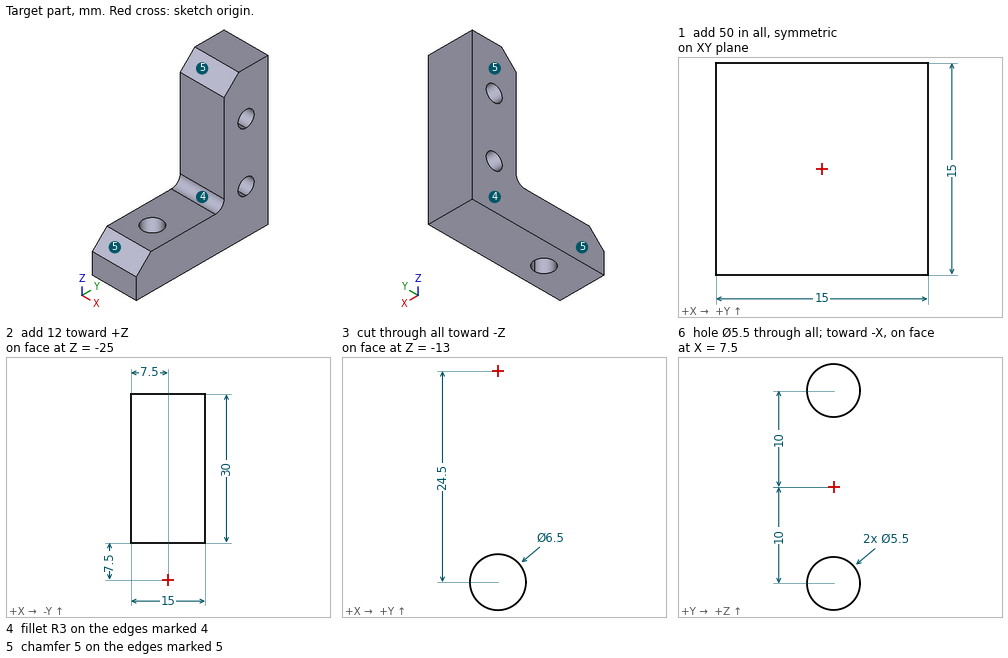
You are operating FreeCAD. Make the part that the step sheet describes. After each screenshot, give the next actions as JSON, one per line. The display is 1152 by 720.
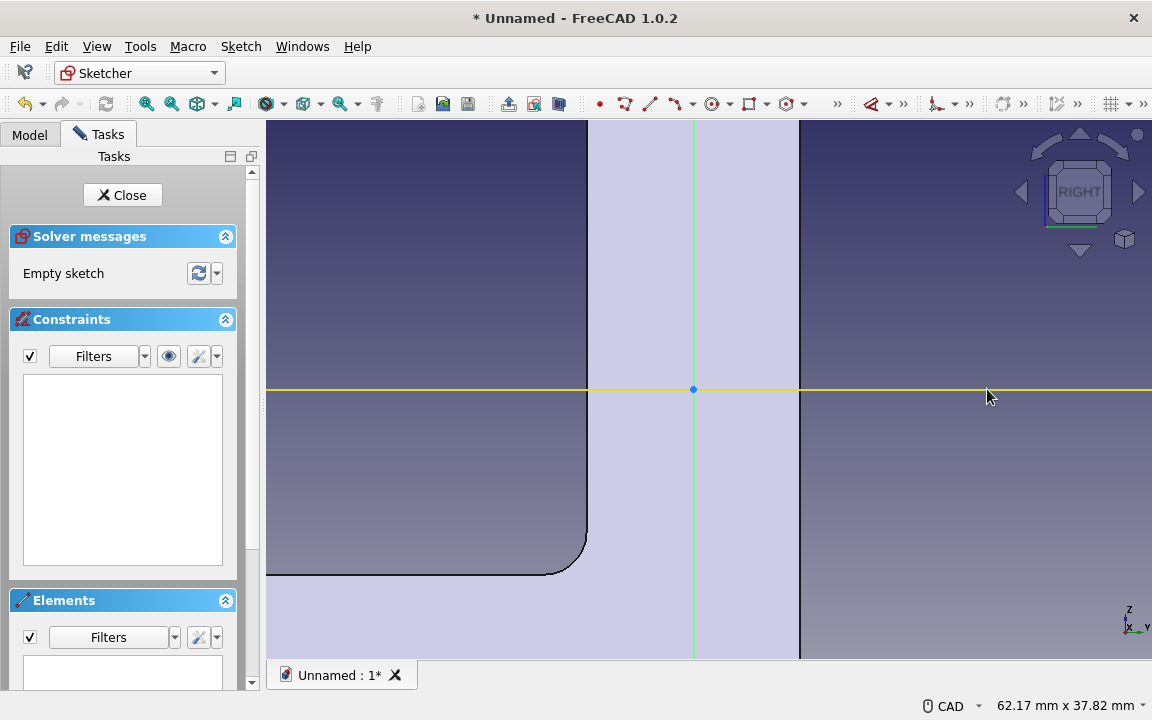
{"action": "key", "text": "g c"}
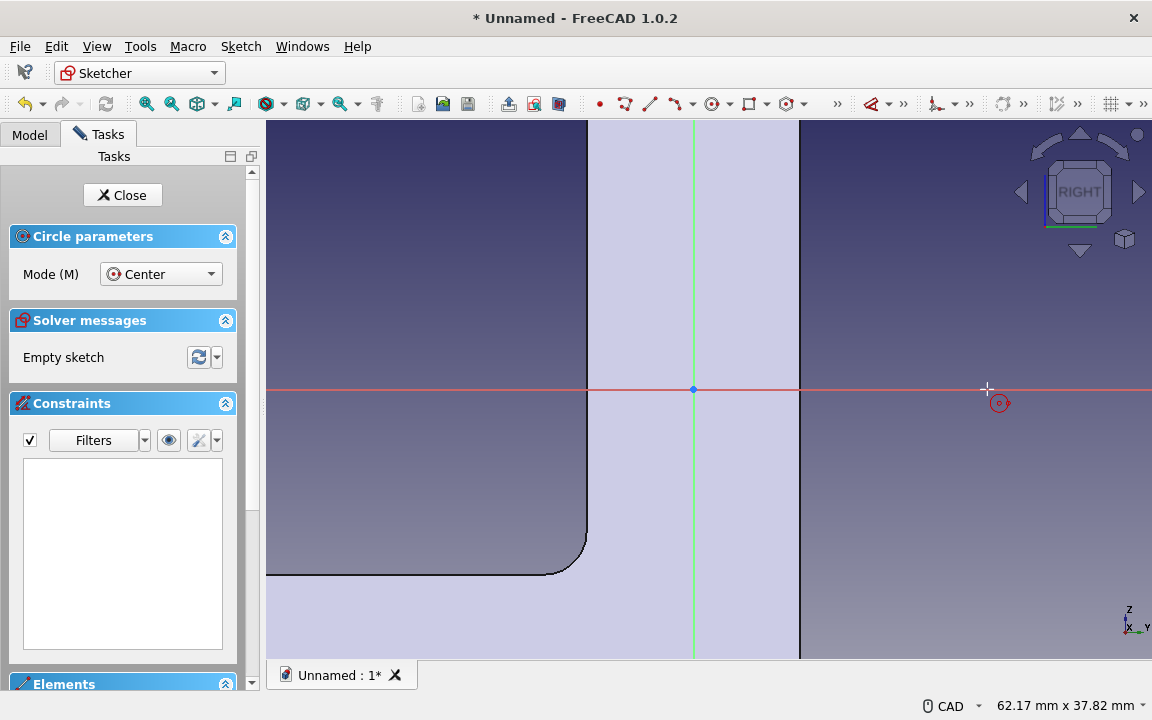
{"action": "left_click", "coordinate": [694, 532]}
{"action": "mouse_move", "coordinate": [721, 504]}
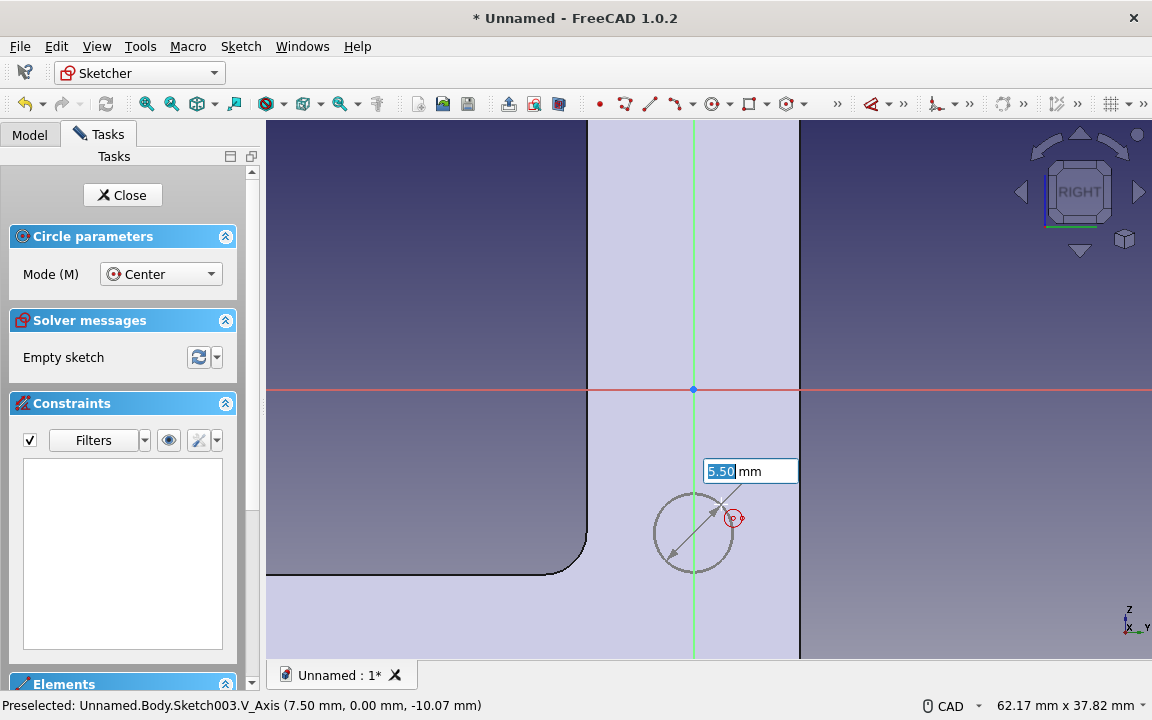
{"action": "type", "text": "5.5"}
{"action": "key", "text": "Return"}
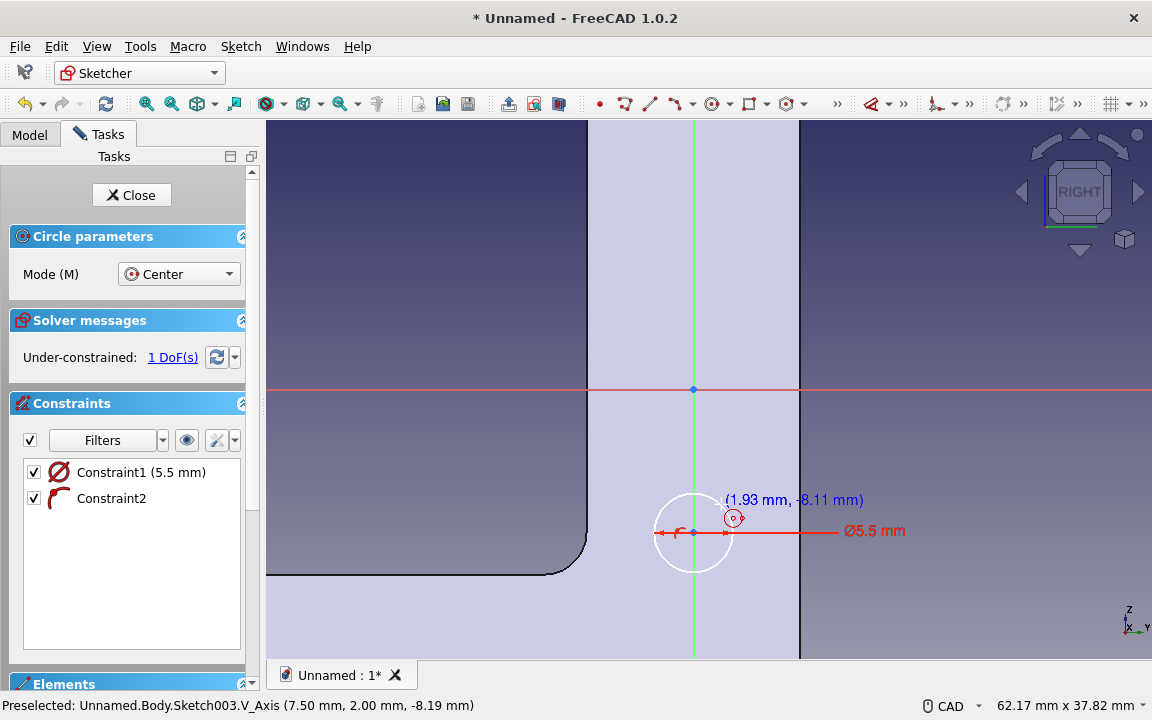
{"action": "left_click", "coordinate": [694, 247]}
{"action": "mouse_move", "coordinate": [721, 219]}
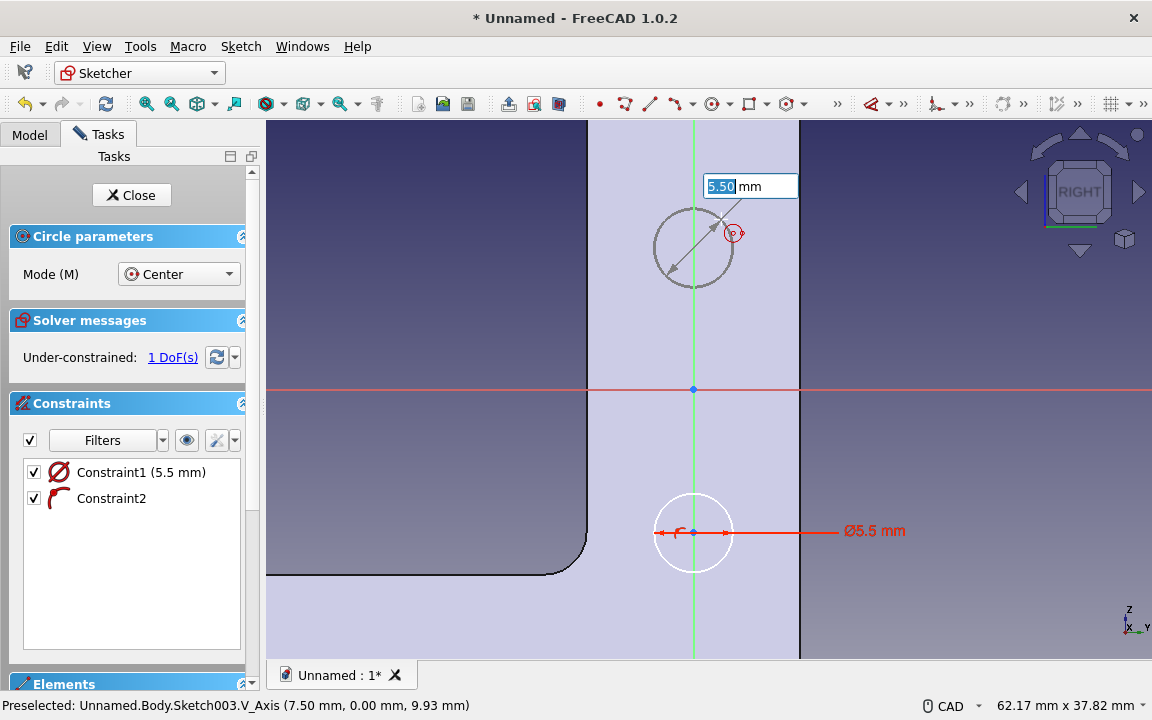
{"action": "type", "text": "5.5"}
{"action": "key", "text": "Return"}
{"action": "key", "text": "Escape"}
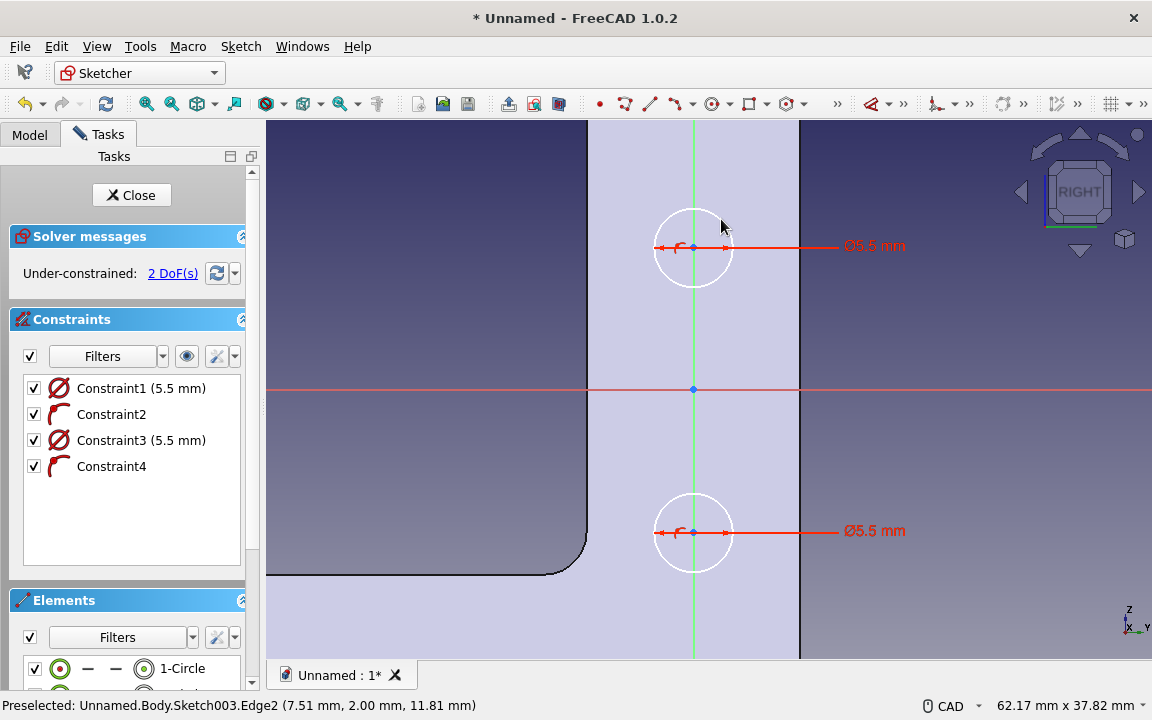
{"action": "left_click", "coordinate": [694, 533]}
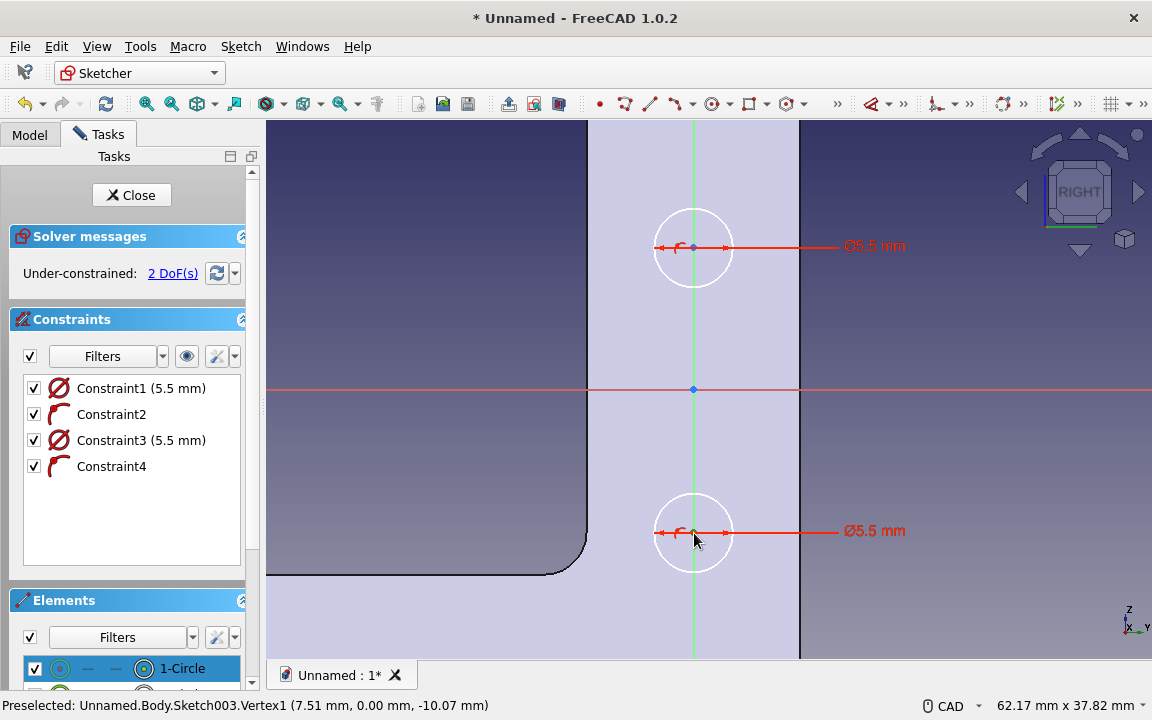
{"action": "key", "text": "i"}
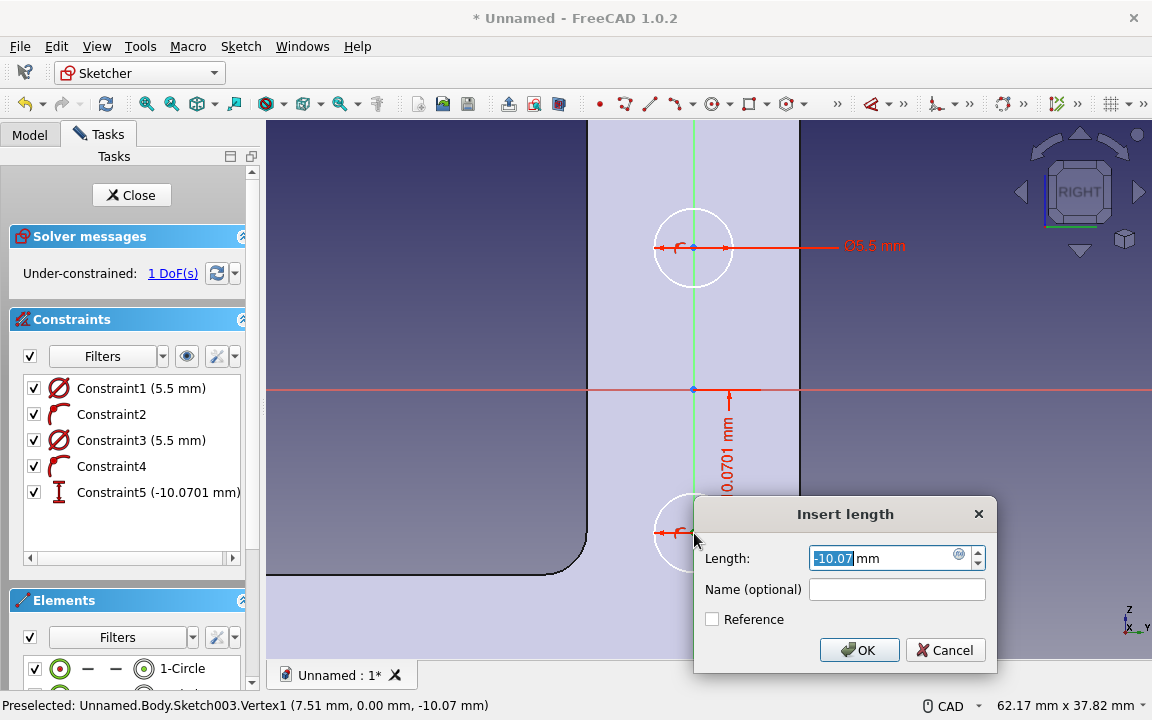
{"action": "type", "text": "-10"}
{"action": "key", "text": "Return"}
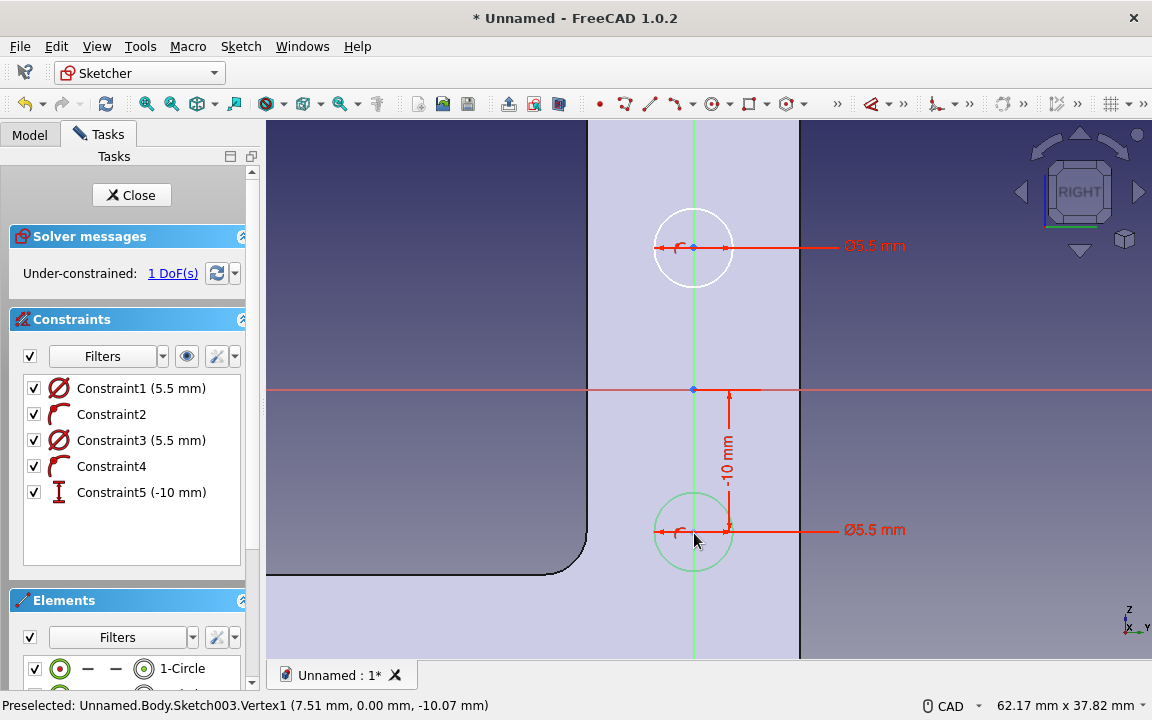
{"action": "left_click", "coordinate": [694, 248]}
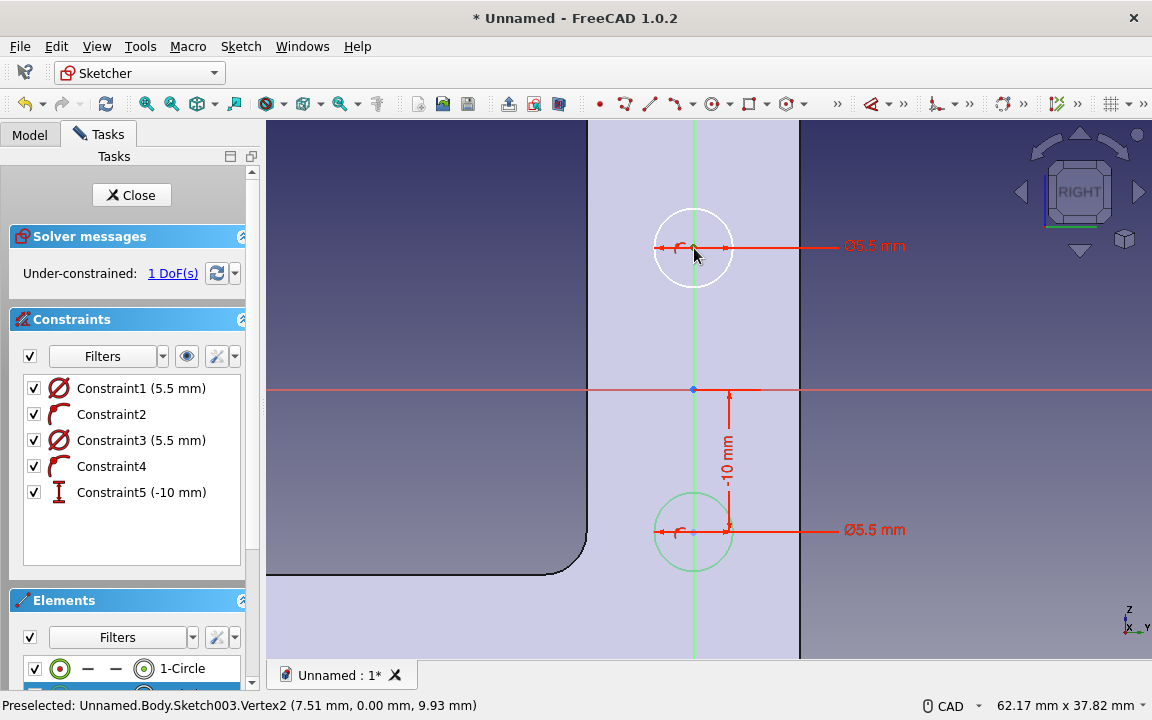
{"action": "left_click", "coordinate": [888, 104]}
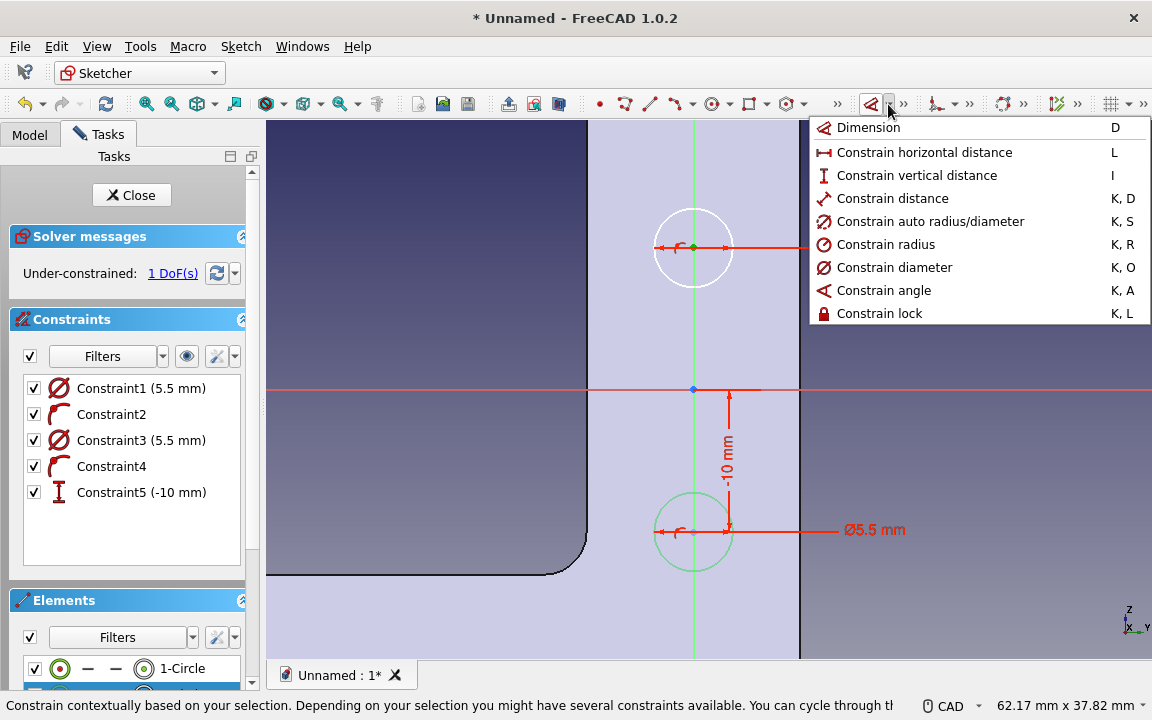
{"action": "left_click", "coordinate": [980, 176]}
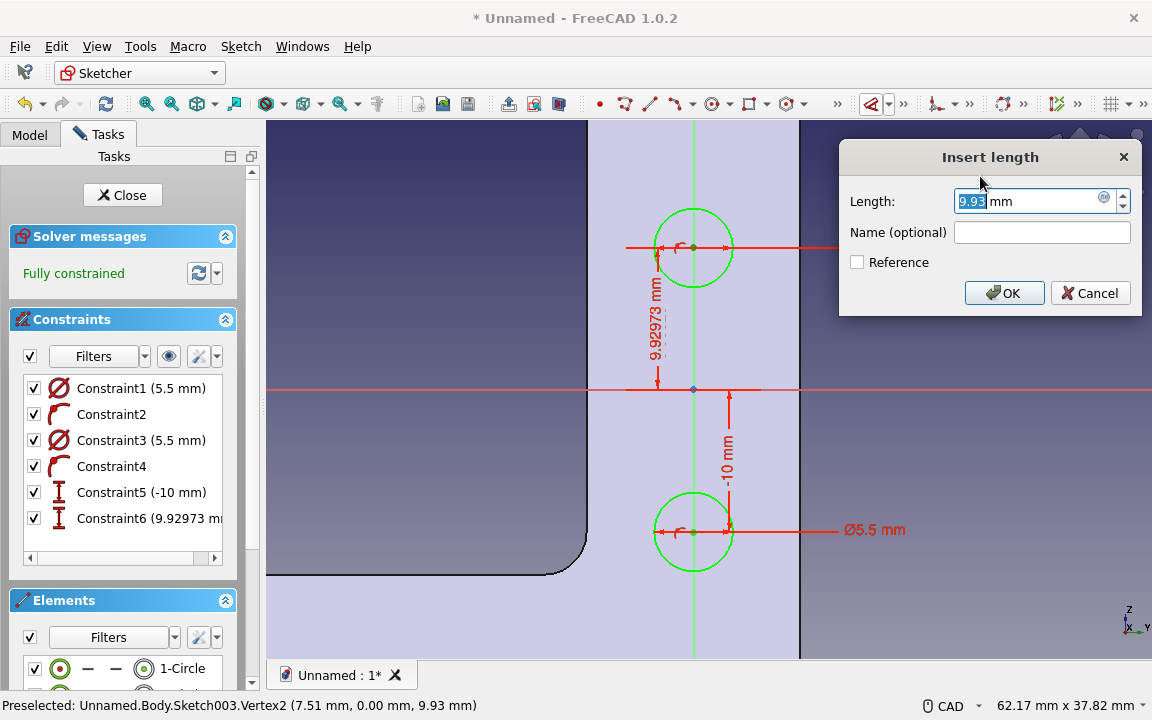
{"action": "type", "text": "10"}
{"action": "key", "text": "Return"}